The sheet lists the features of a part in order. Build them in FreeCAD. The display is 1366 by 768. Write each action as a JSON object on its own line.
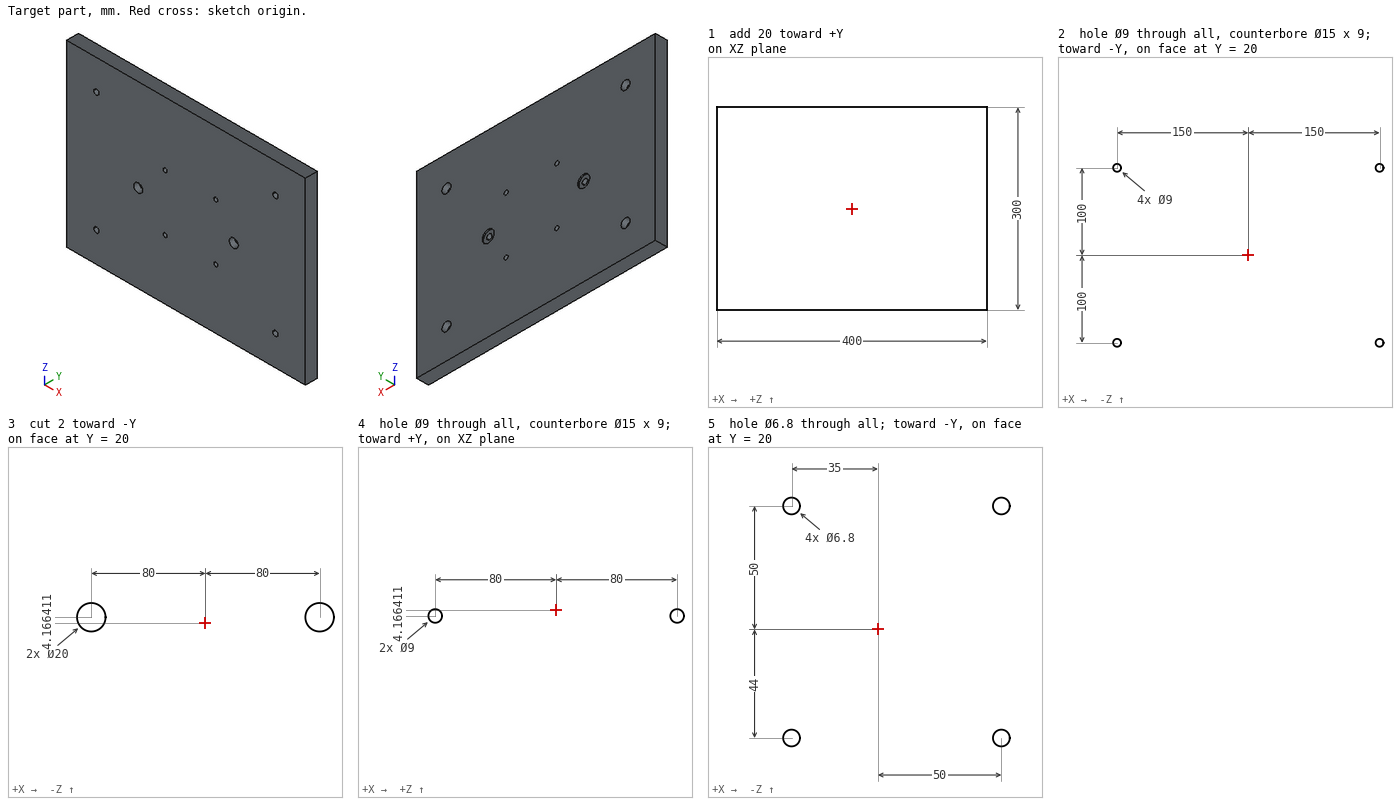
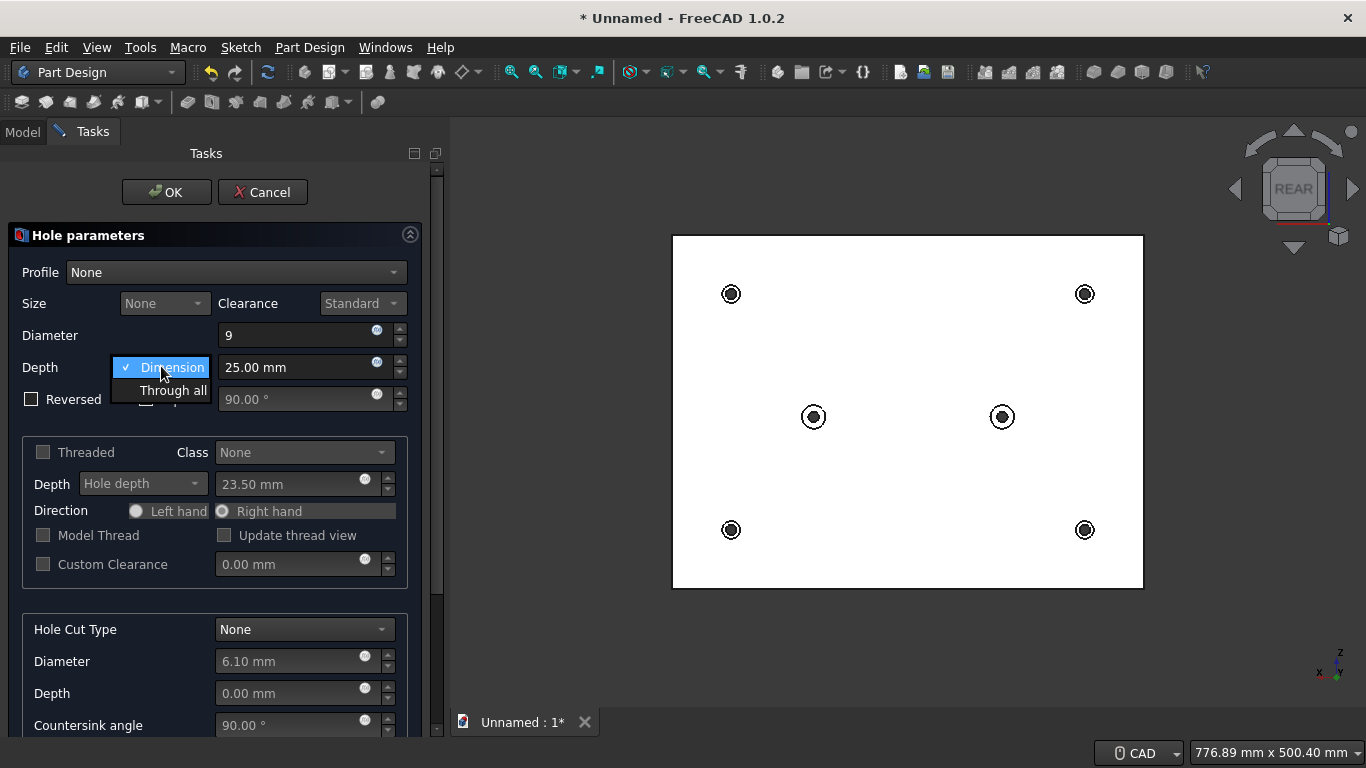
{"action": "left_click", "coordinate": [160, 390]}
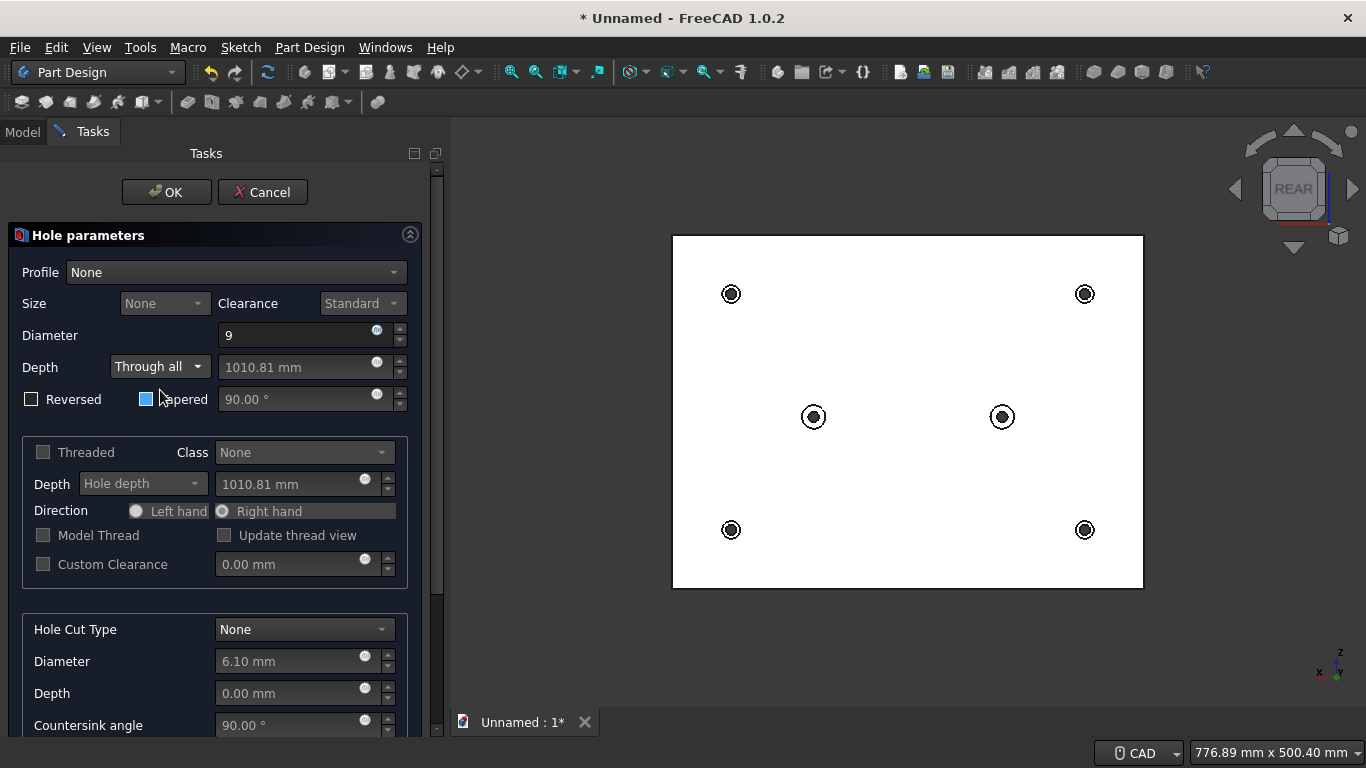
{"action": "left_click", "coordinate": [306, 630]}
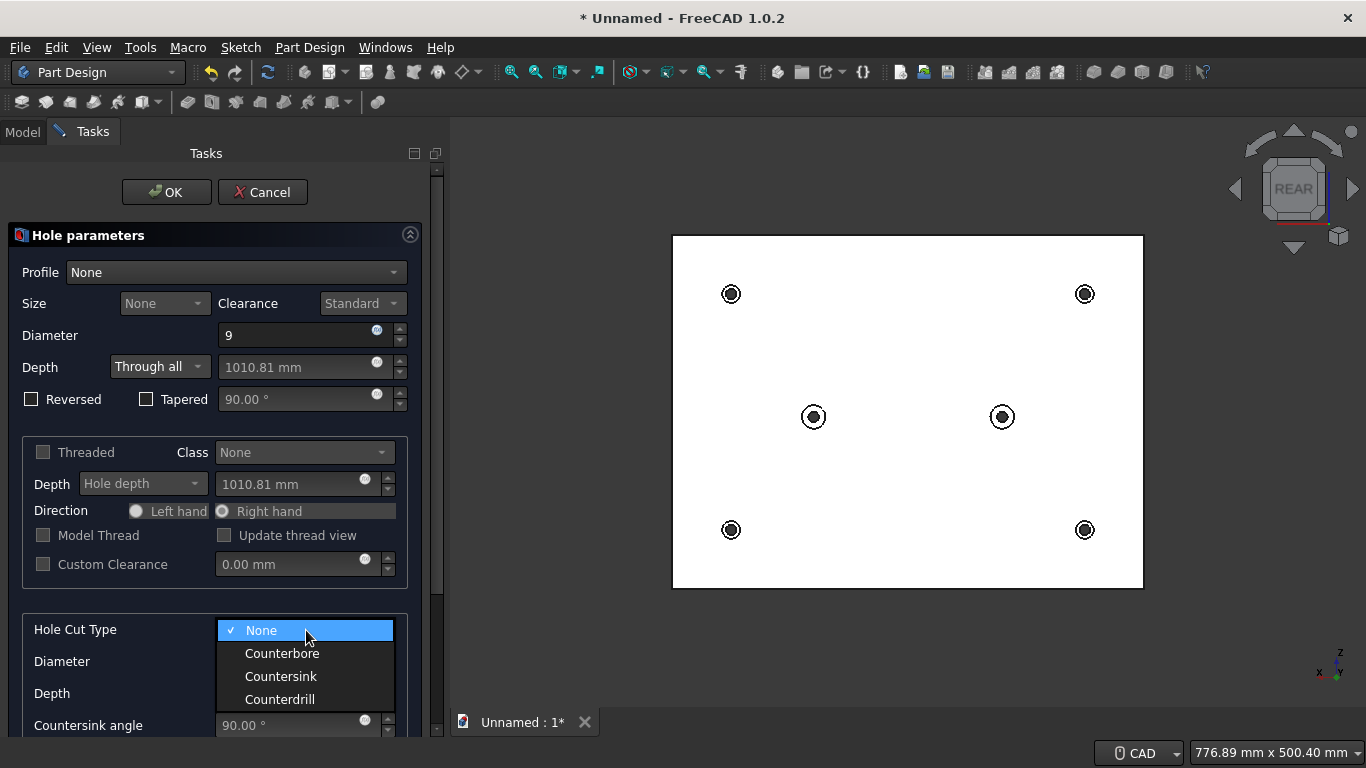
{"action": "left_click", "coordinate": [304, 654]}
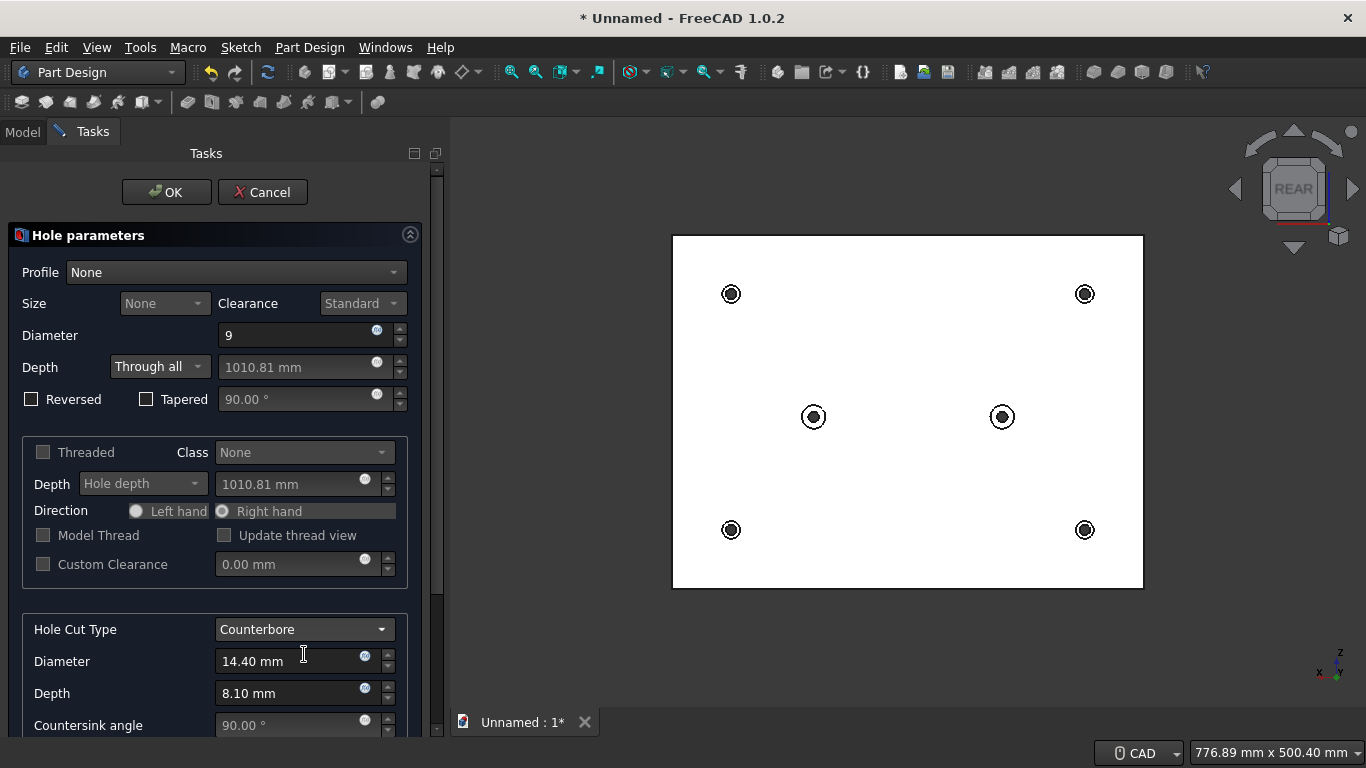
{"action": "triple_click", "coordinate": [298, 661]}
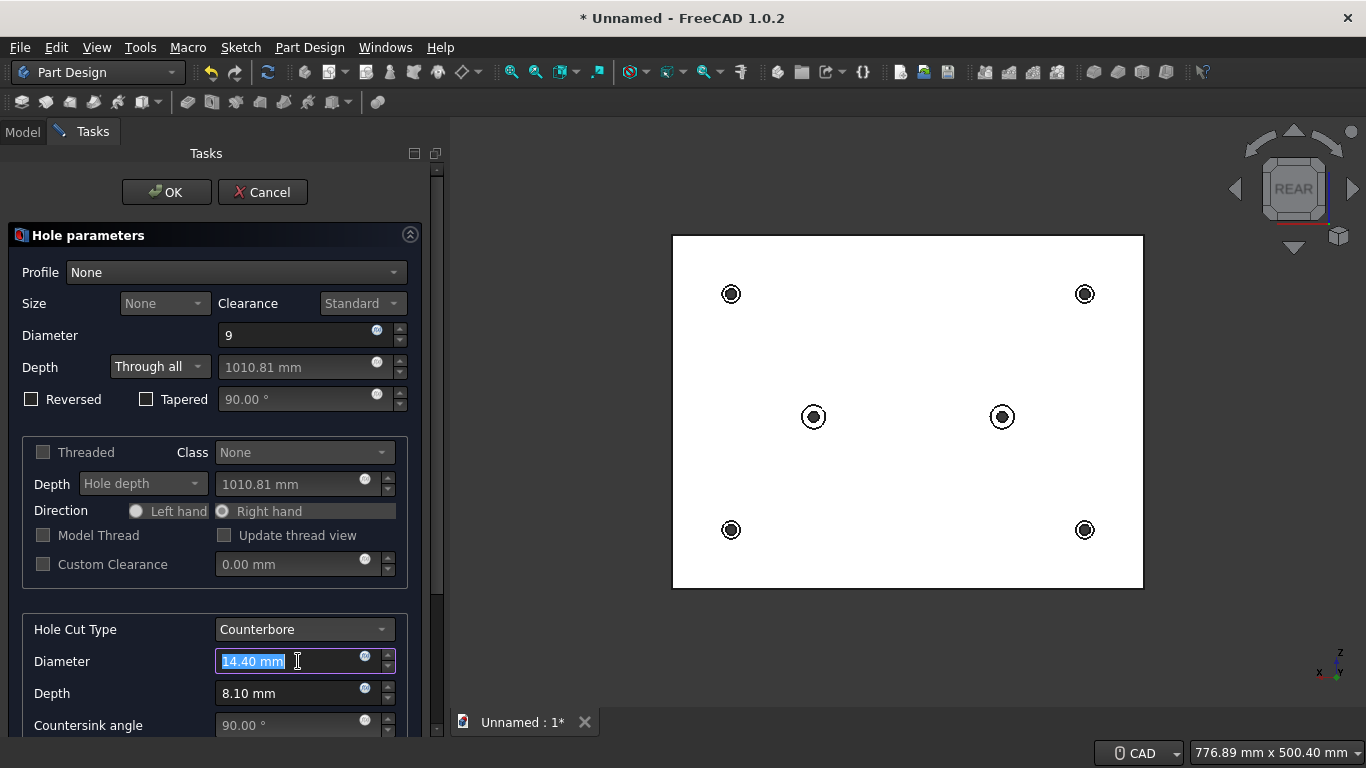
{"action": "type", "text": "15"}
{"action": "key", "text": "Tab"}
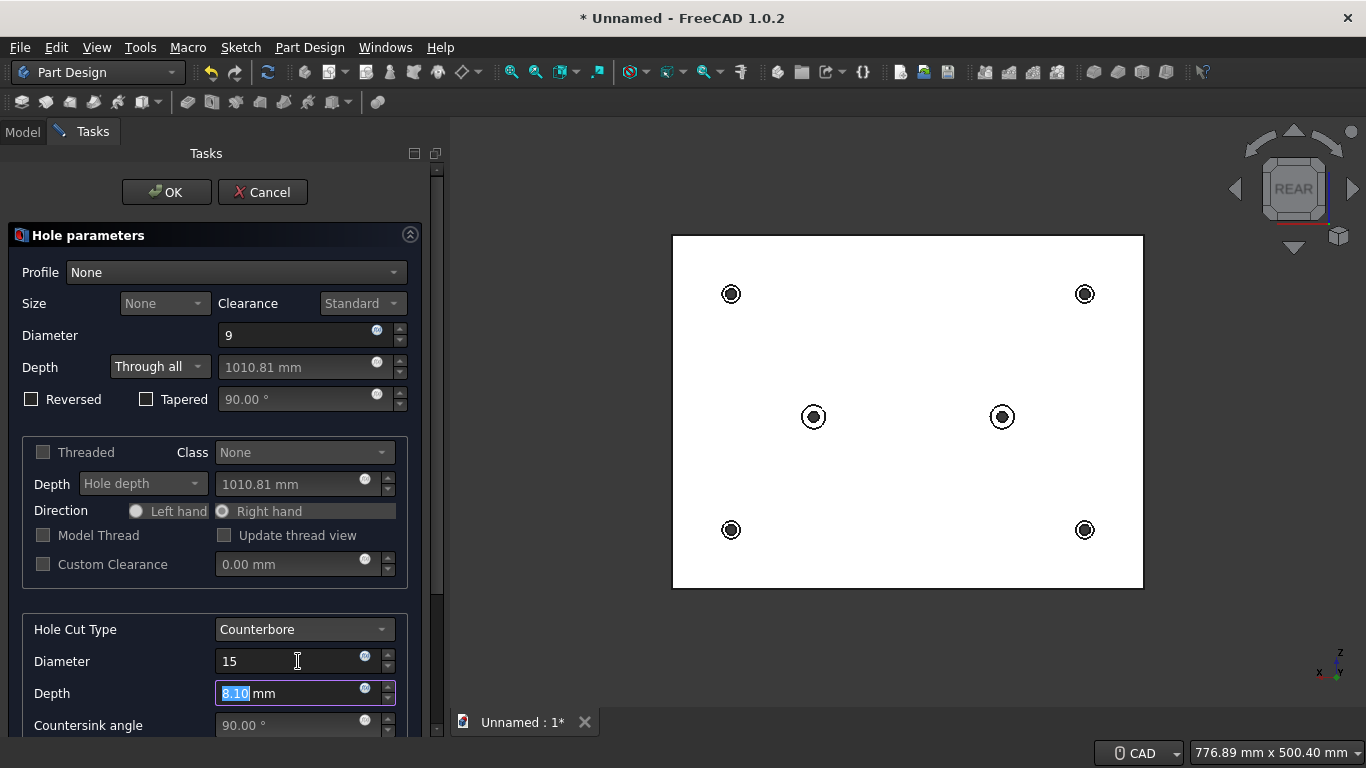
{"action": "type", "text": "9"}
{"action": "key", "text": "Tab"}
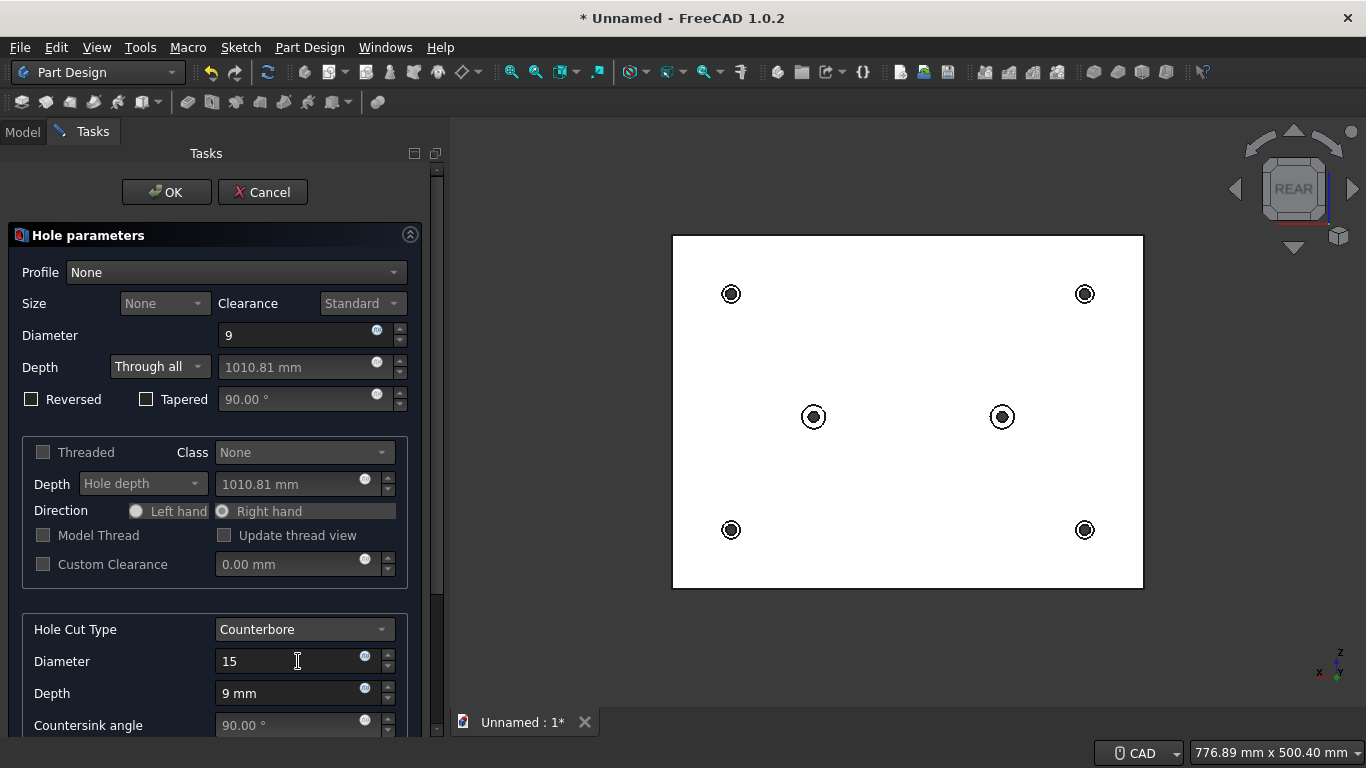
{"action": "left_click", "coordinate": [167, 192]}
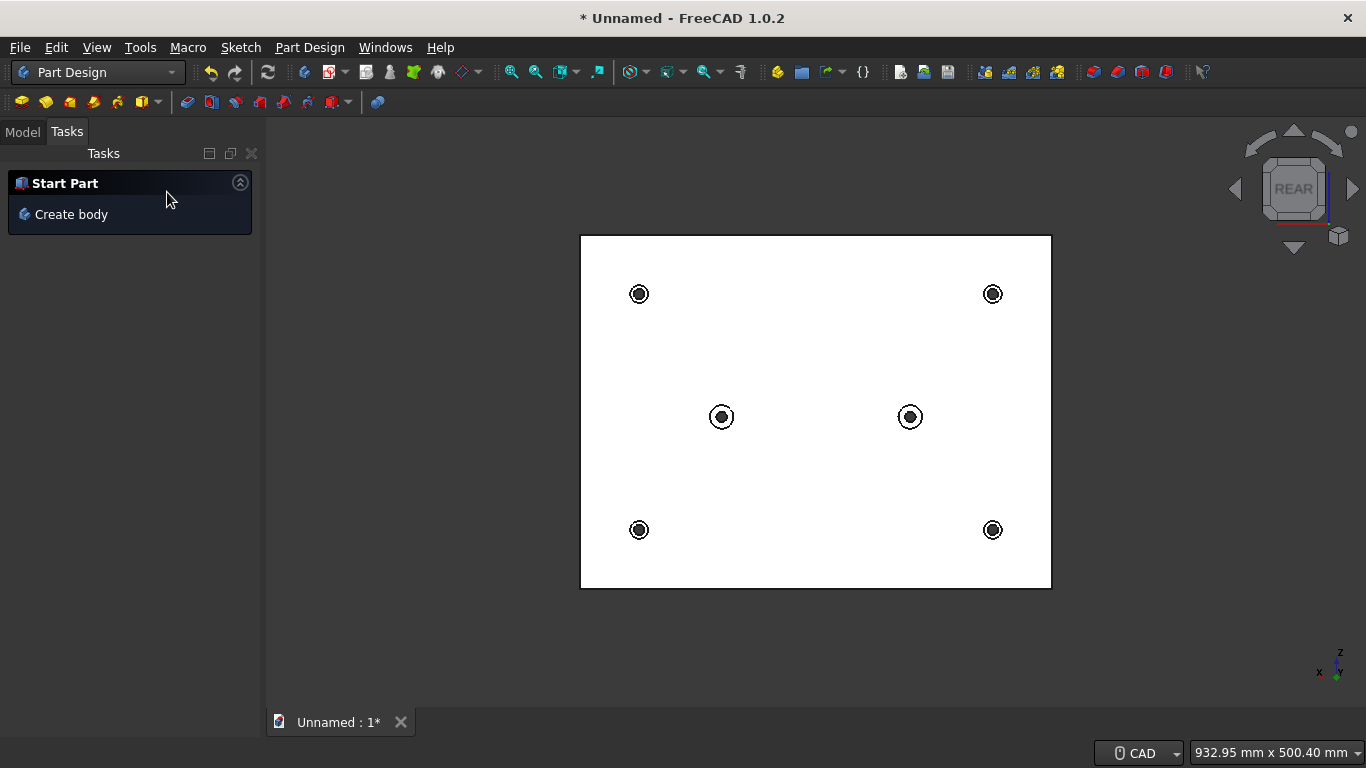
{"action": "left_click", "coordinate": [816, 360]}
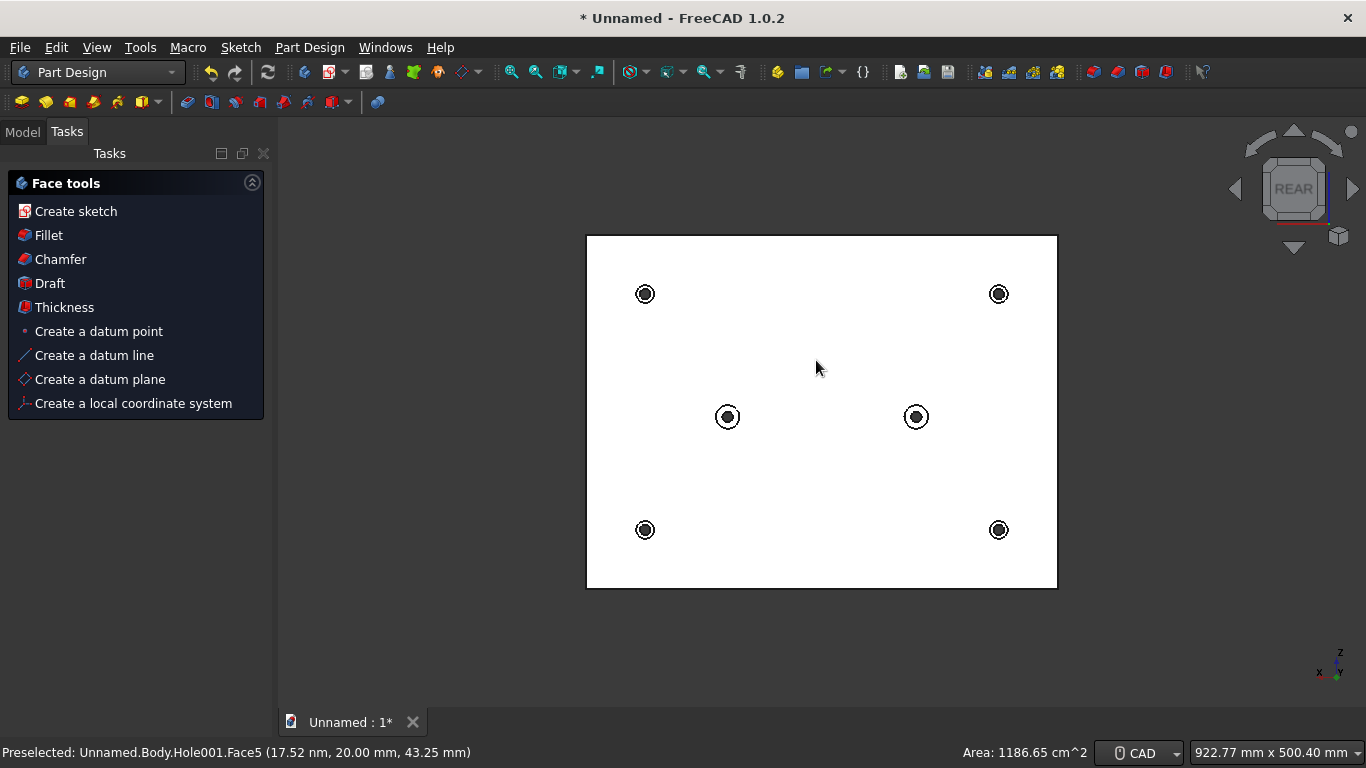
{"action": "left_click", "coordinate": [330, 72]}